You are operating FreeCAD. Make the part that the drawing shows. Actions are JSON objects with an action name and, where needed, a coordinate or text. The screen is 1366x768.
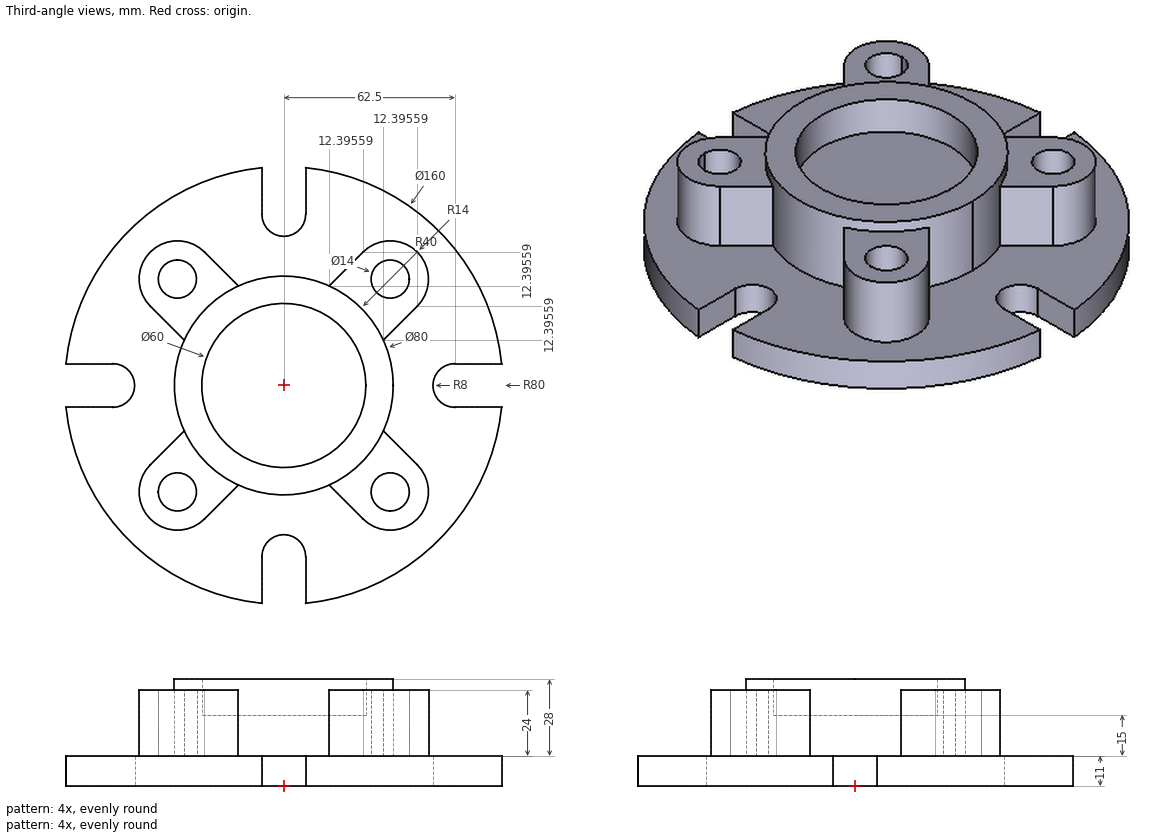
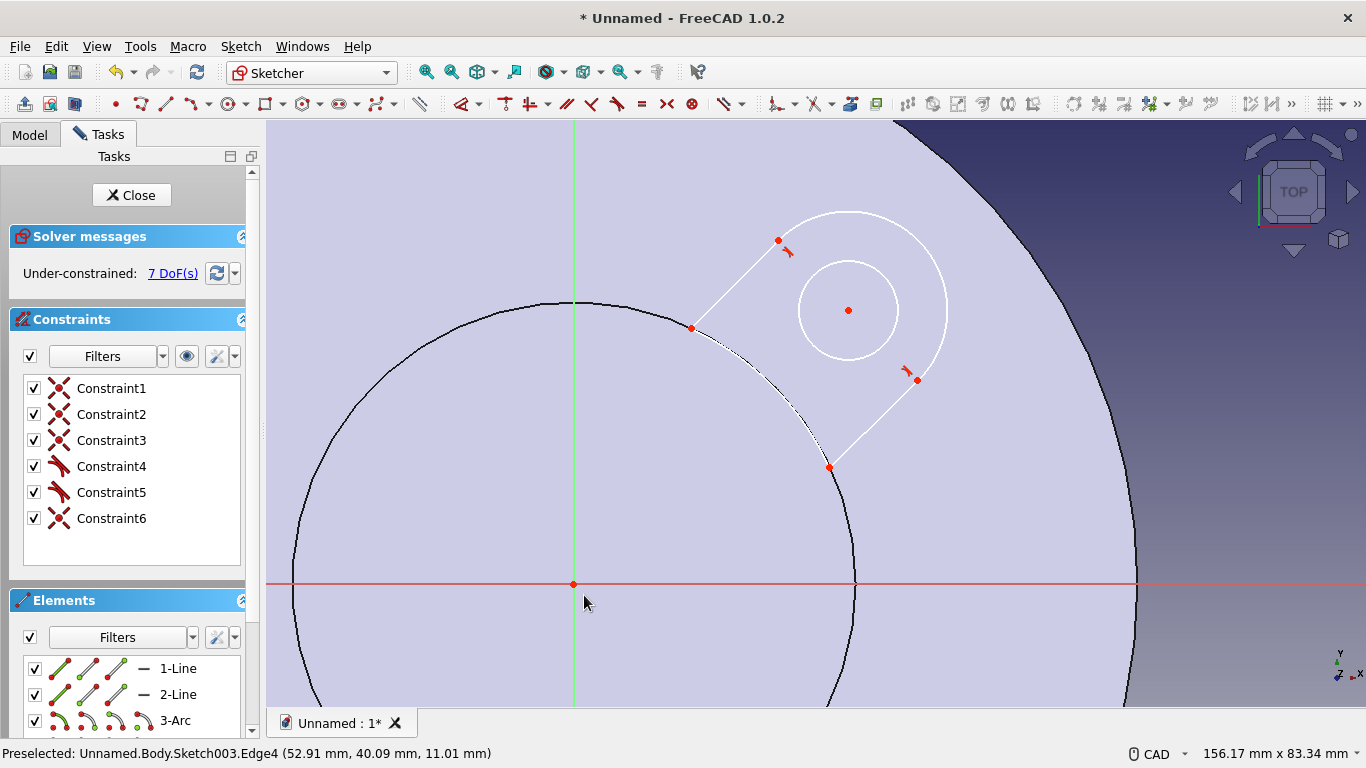
{"action": "key", "text": "d"}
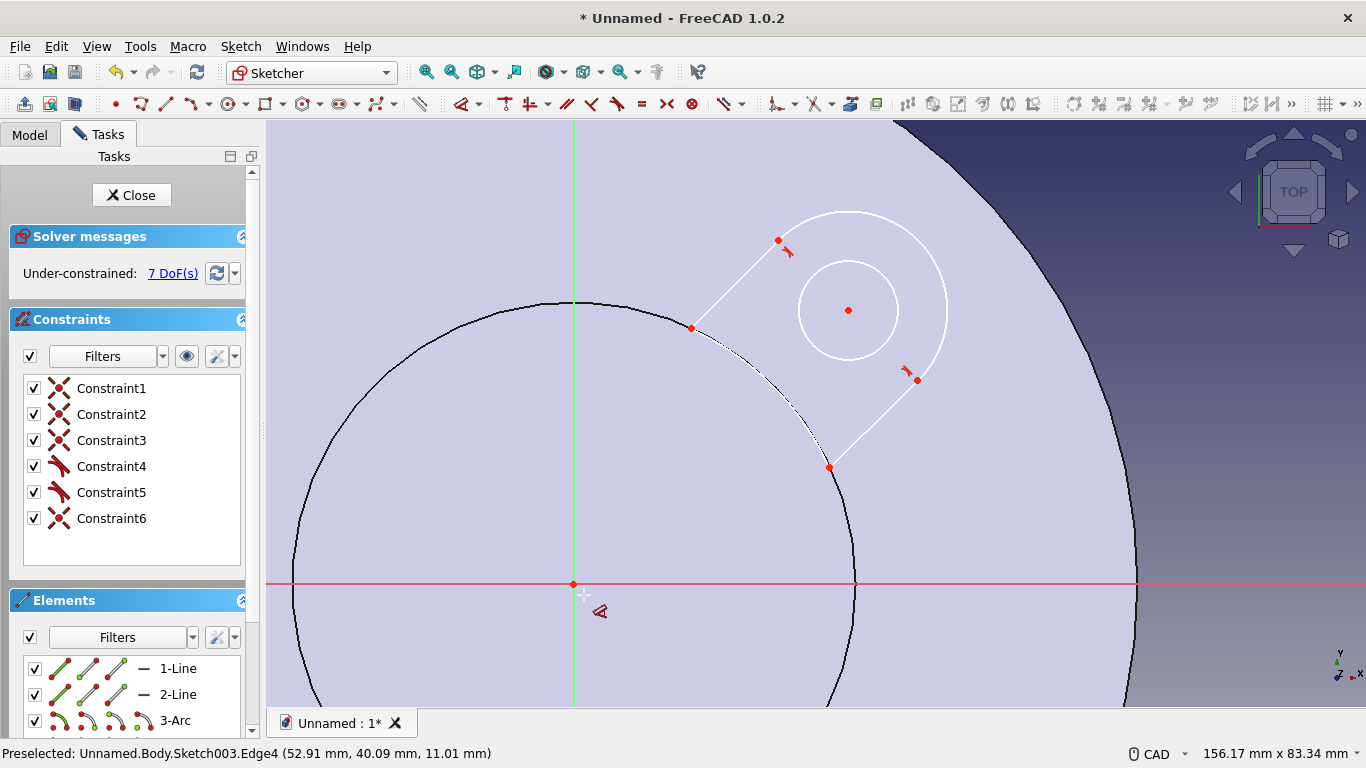
{"action": "left_click", "coordinate": [799, 416]}
{"action": "left_click", "coordinate": [825, 397]}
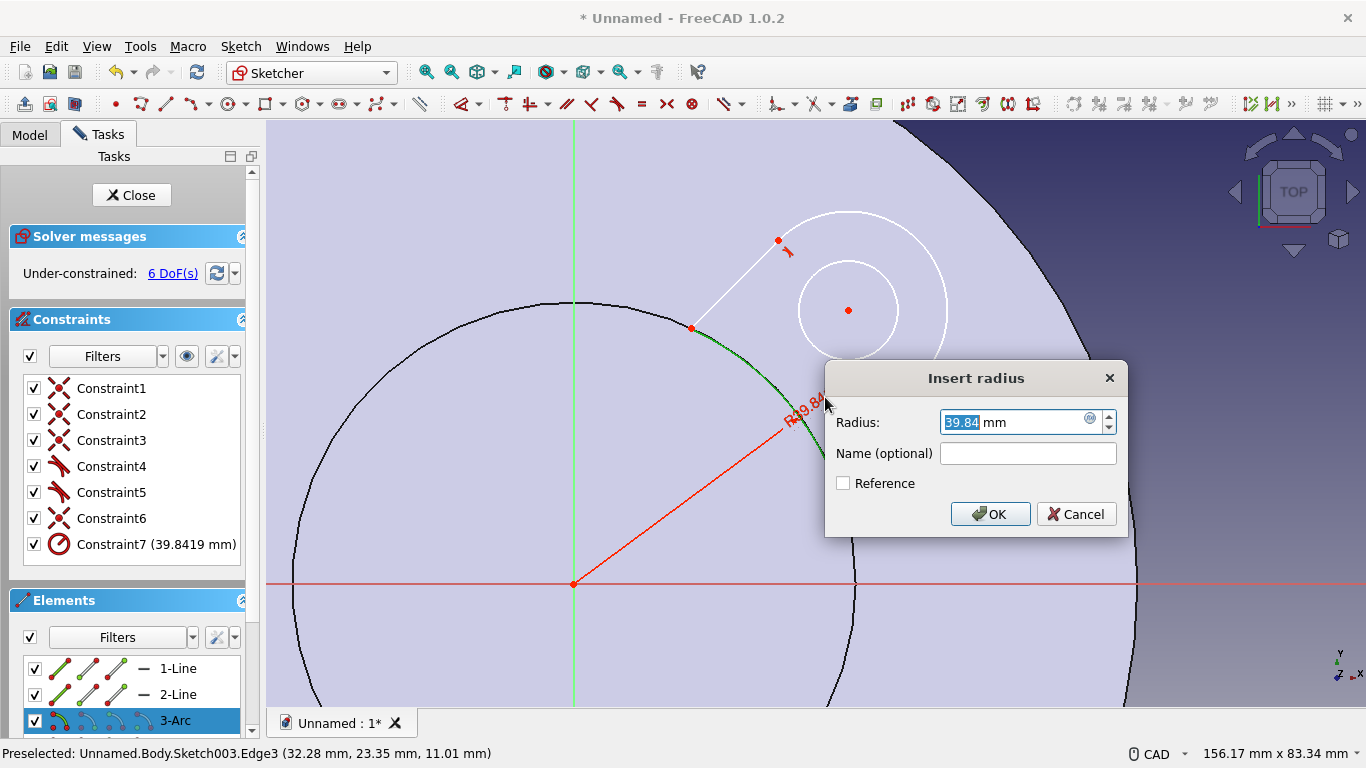
{"action": "type", "text": "40"}
{"action": "key", "text": "Return"}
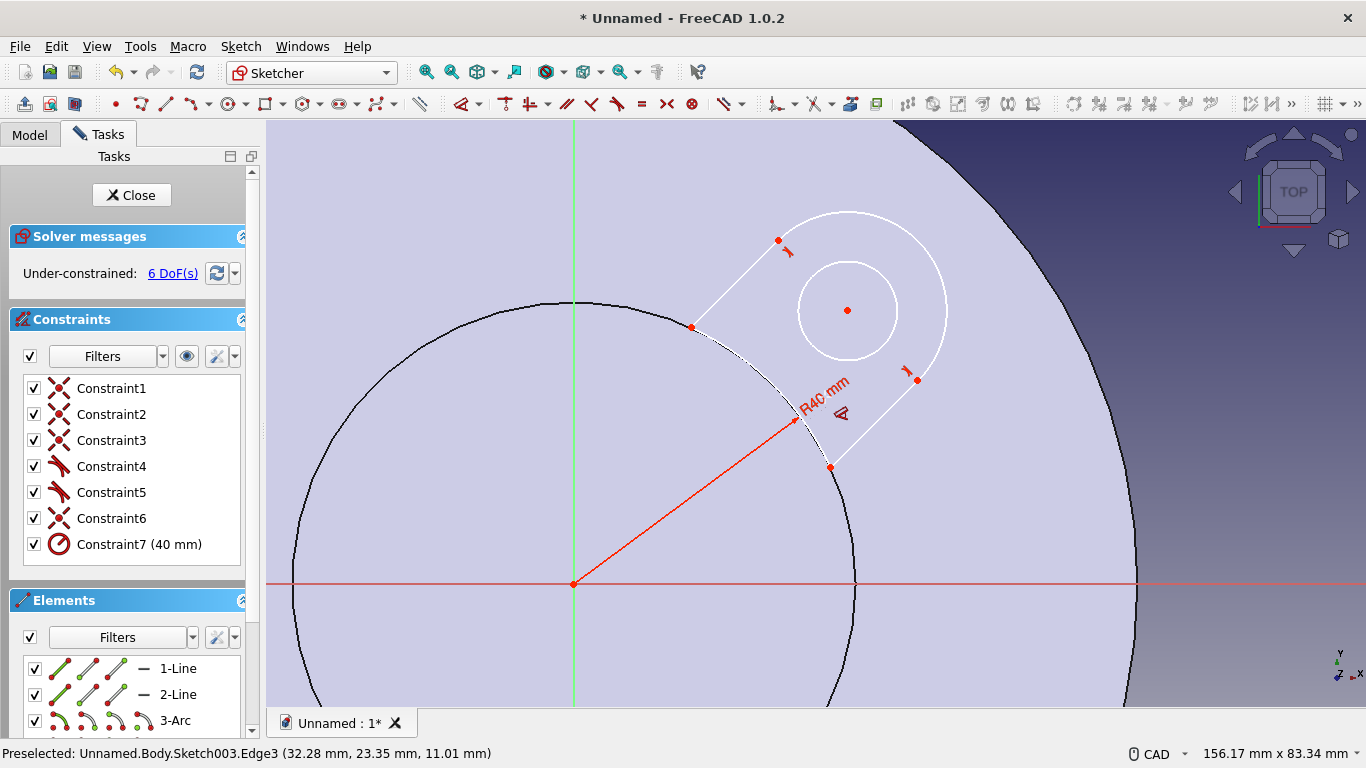
{"action": "left_click", "coordinate": [946, 296]}
{"action": "left_click", "coordinate": [978, 291]}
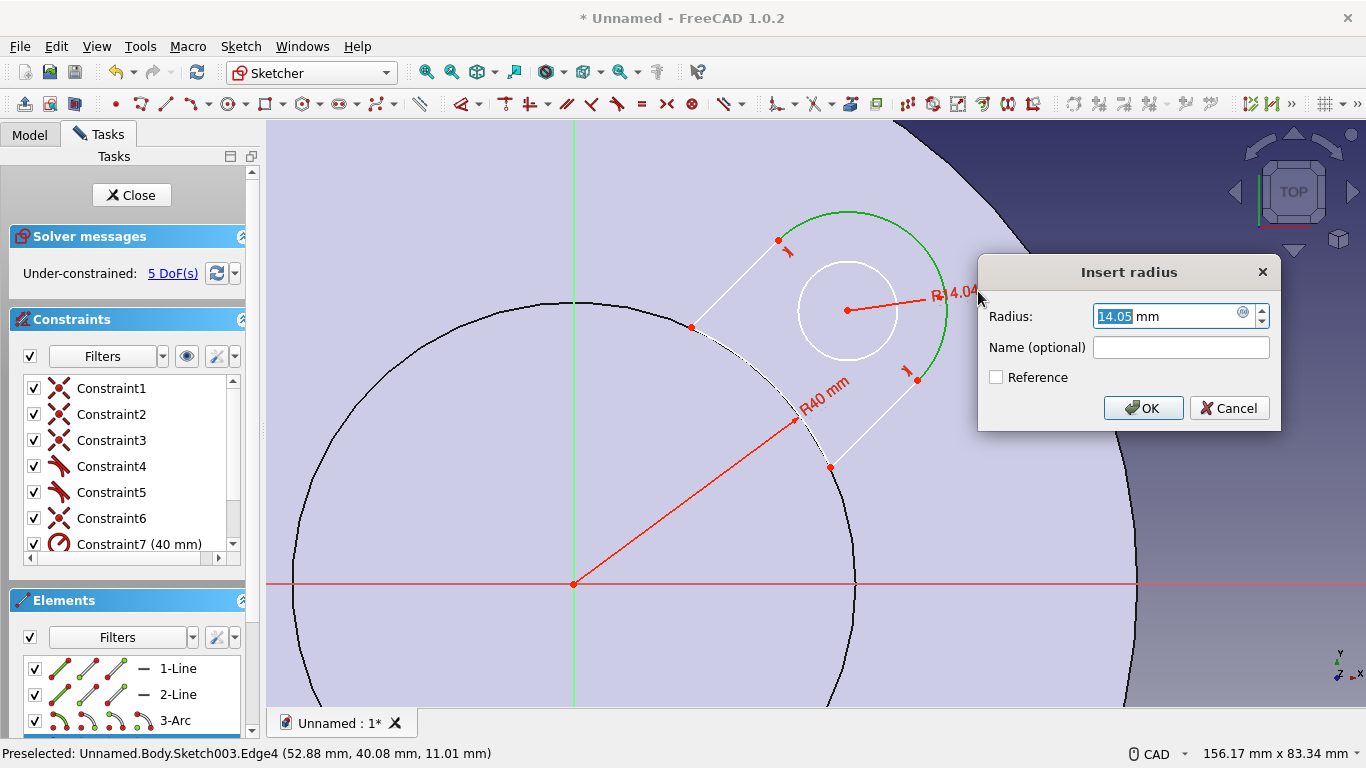
{"action": "type", "text": "14"}
{"action": "key", "text": "Return"}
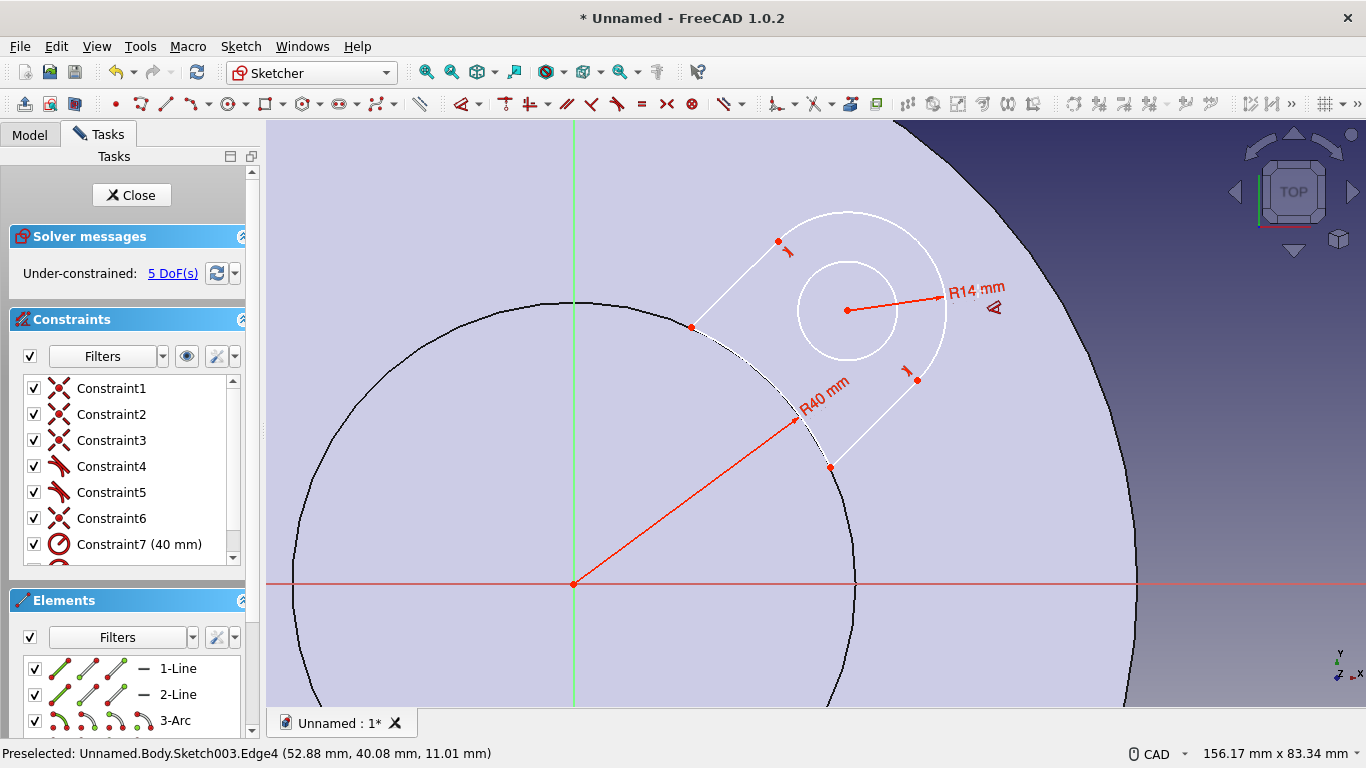
{"action": "left_click", "coordinate": [882, 276]}
{"action": "left_click", "coordinate": [904, 253]}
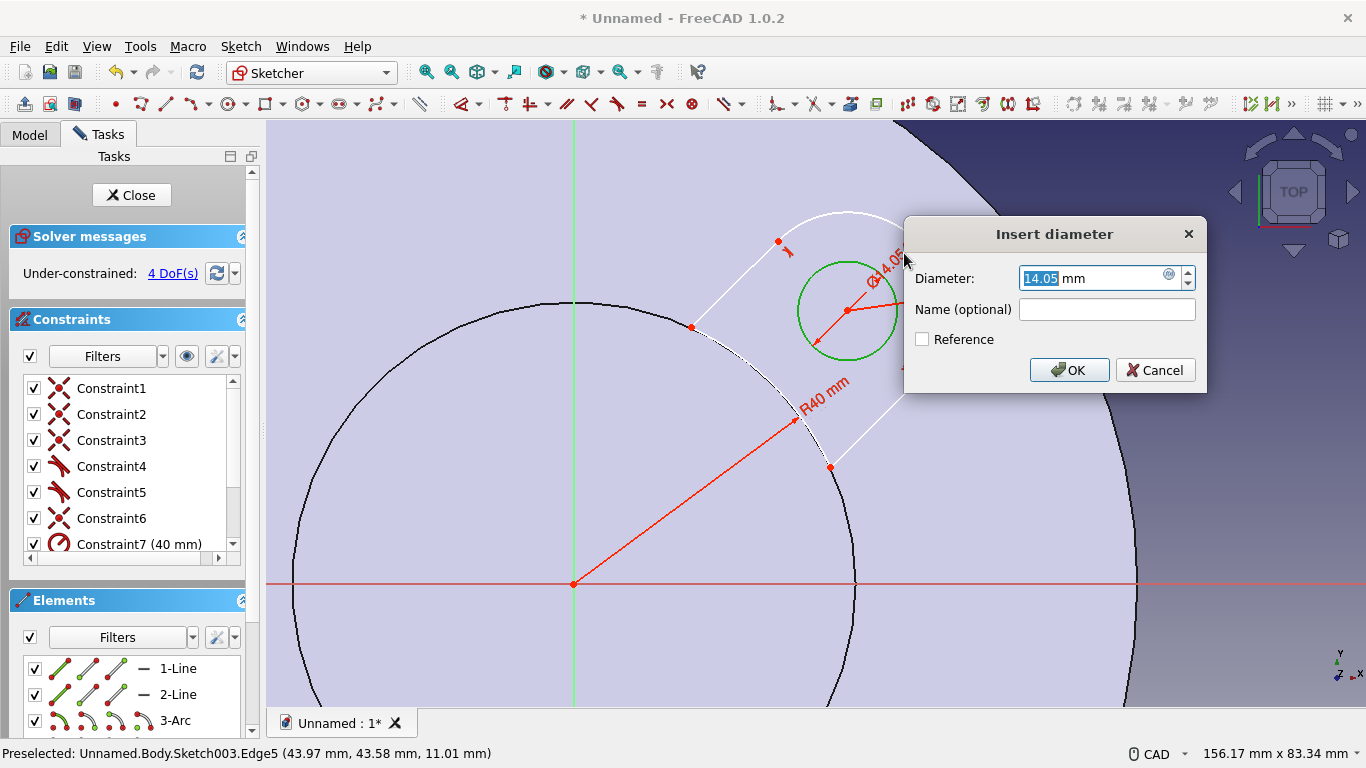
{"action": "type", "text": "14"}
{"action": "key", "text": "Return"}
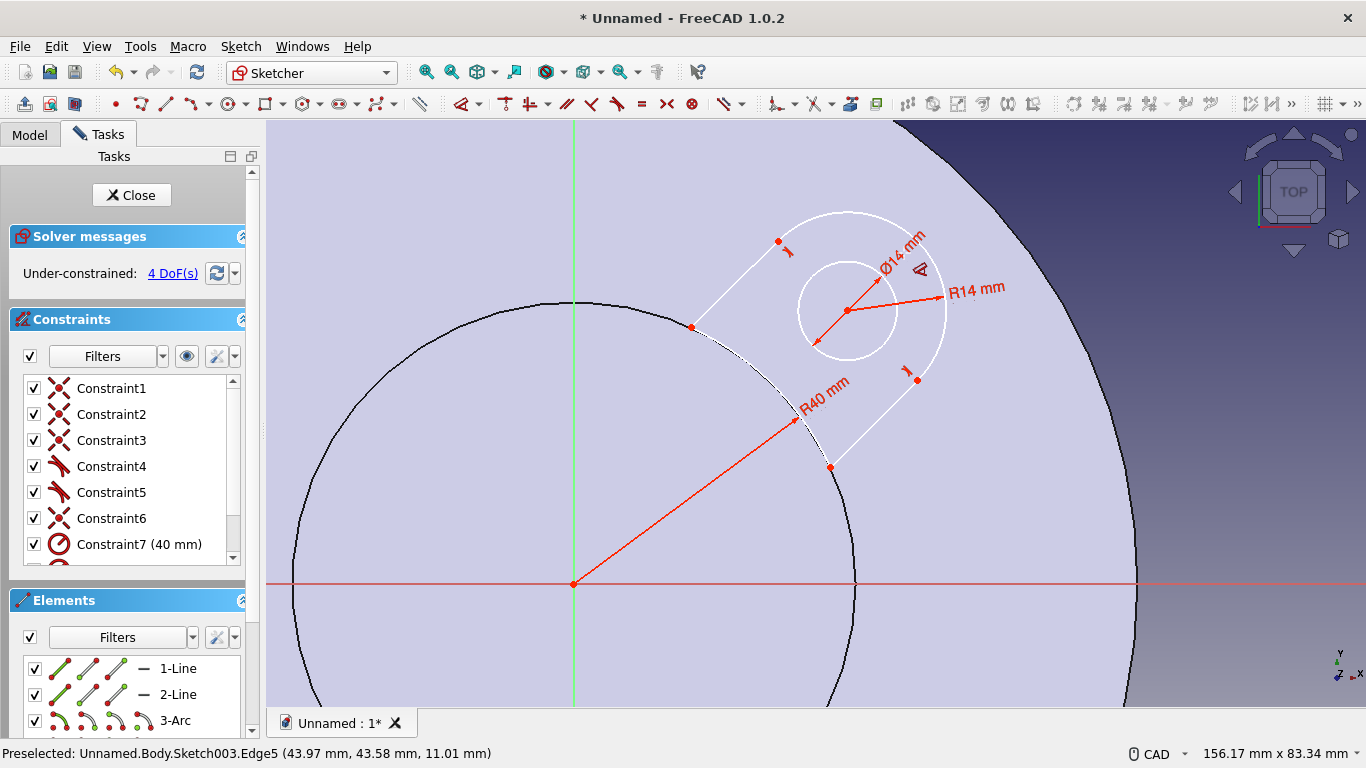
{"action": "left_click", "coordinate": [752, 267]}
{"action": "left_click", "coordinate": [735, 207]}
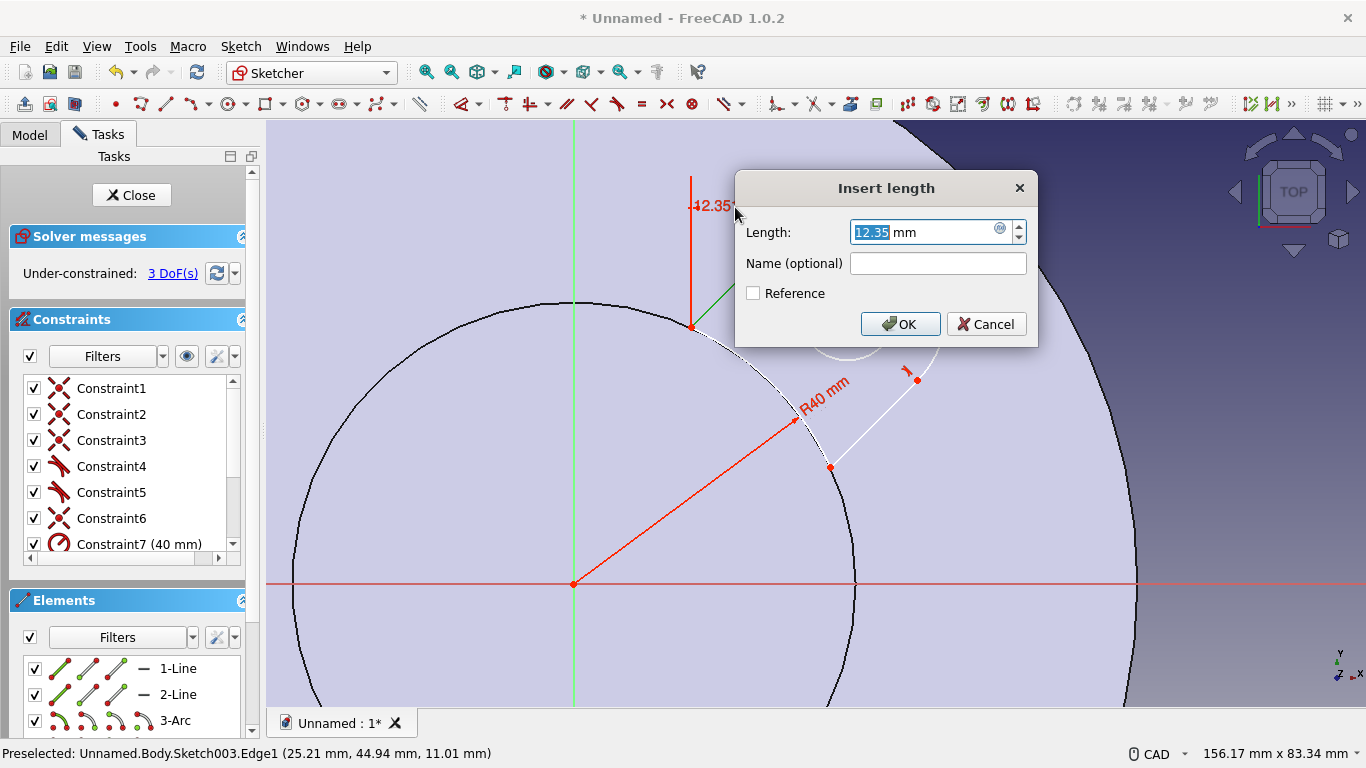
{"action": "type", "text": "12.39559"}
{"action": "key", "text": "Return"}